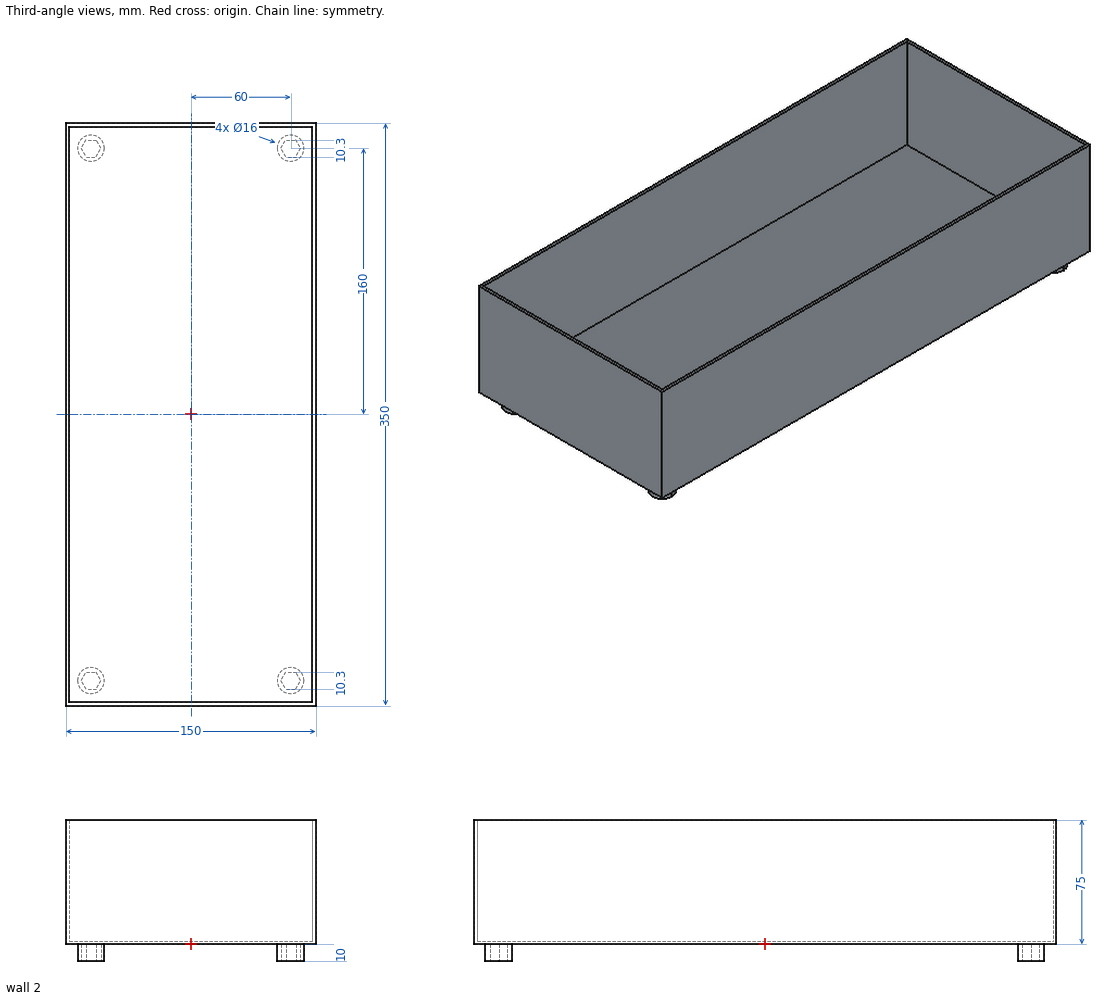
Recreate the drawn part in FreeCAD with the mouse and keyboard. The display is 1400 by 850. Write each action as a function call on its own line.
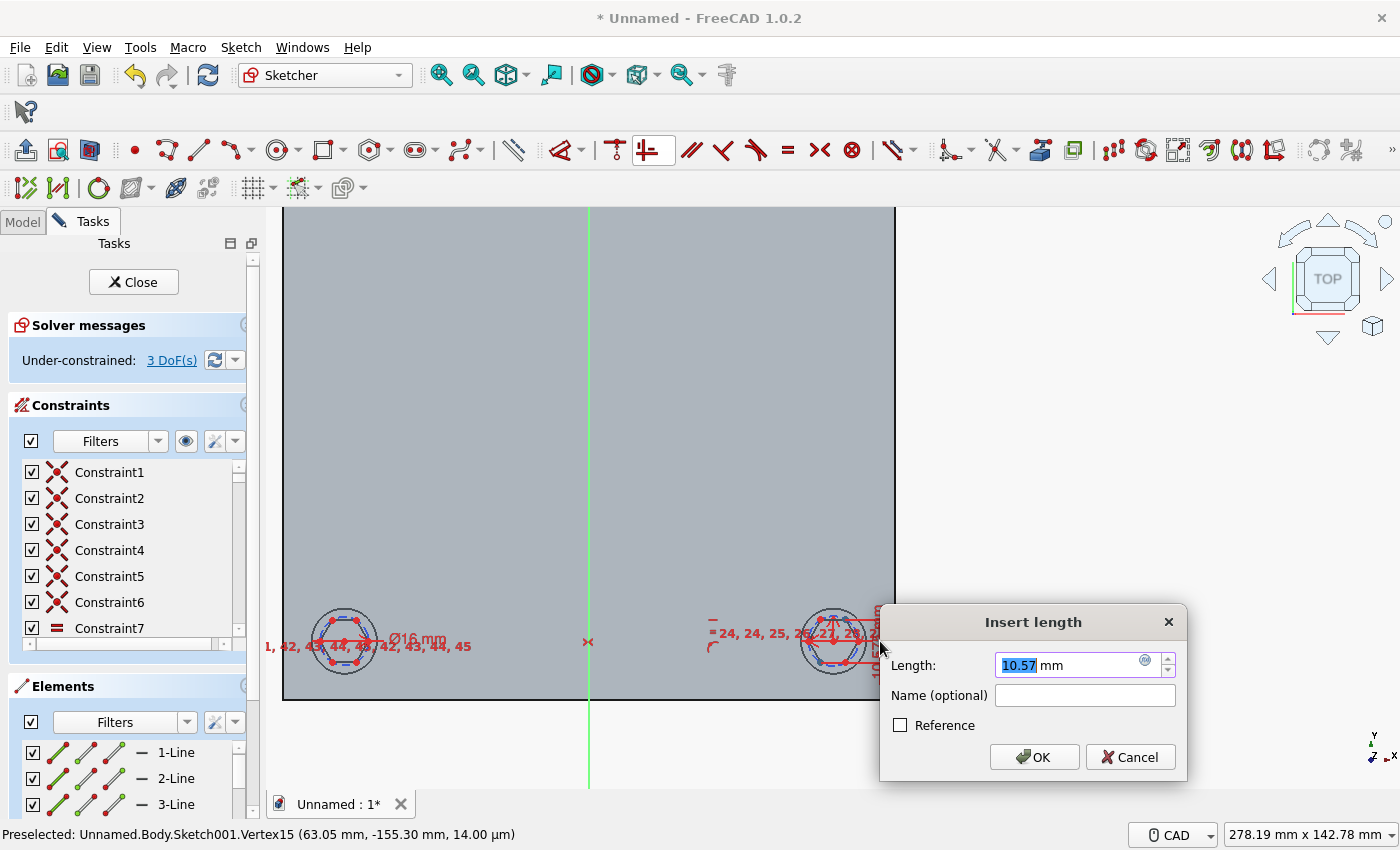
text(10.3)
key(Return)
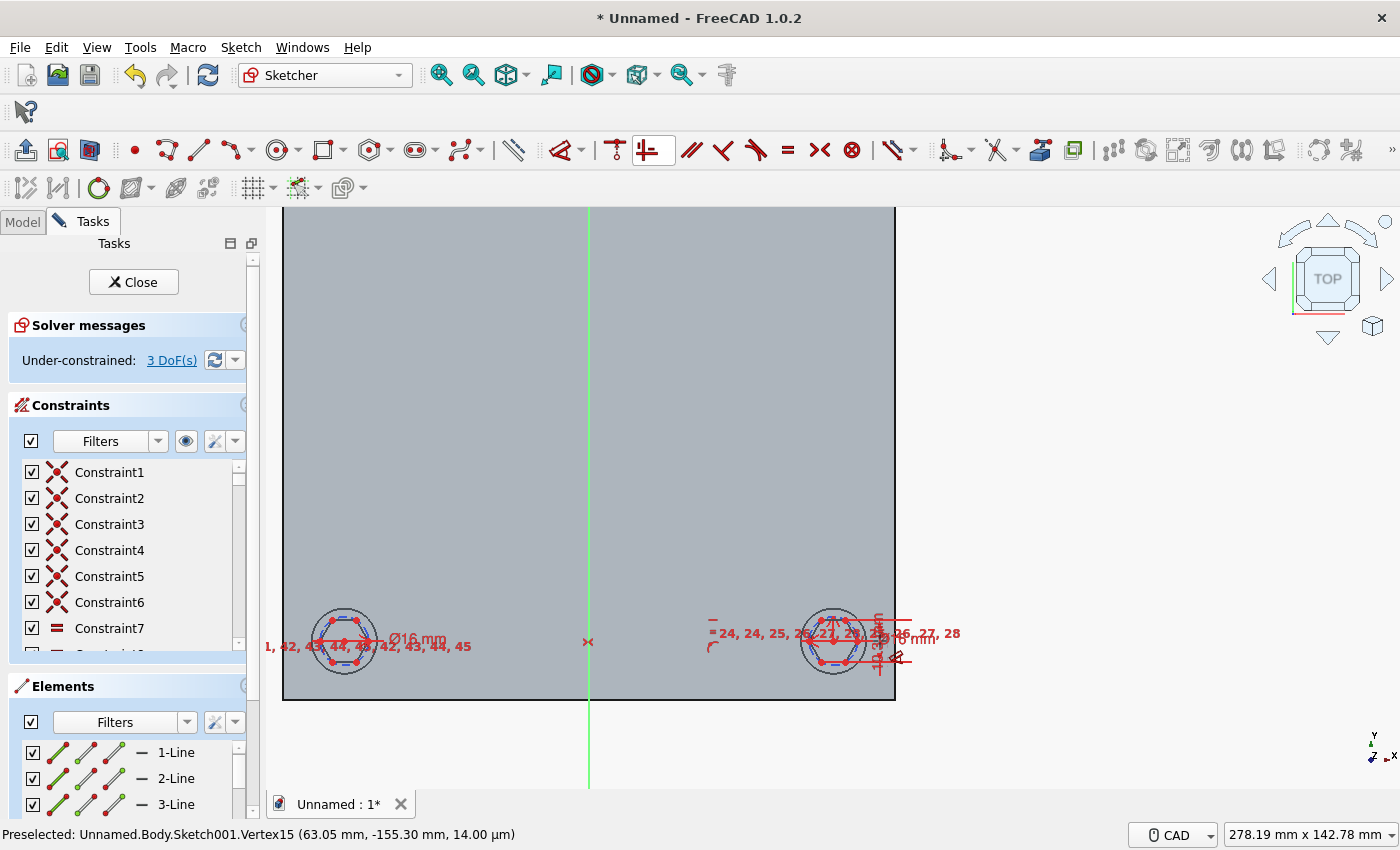
click(332, 662)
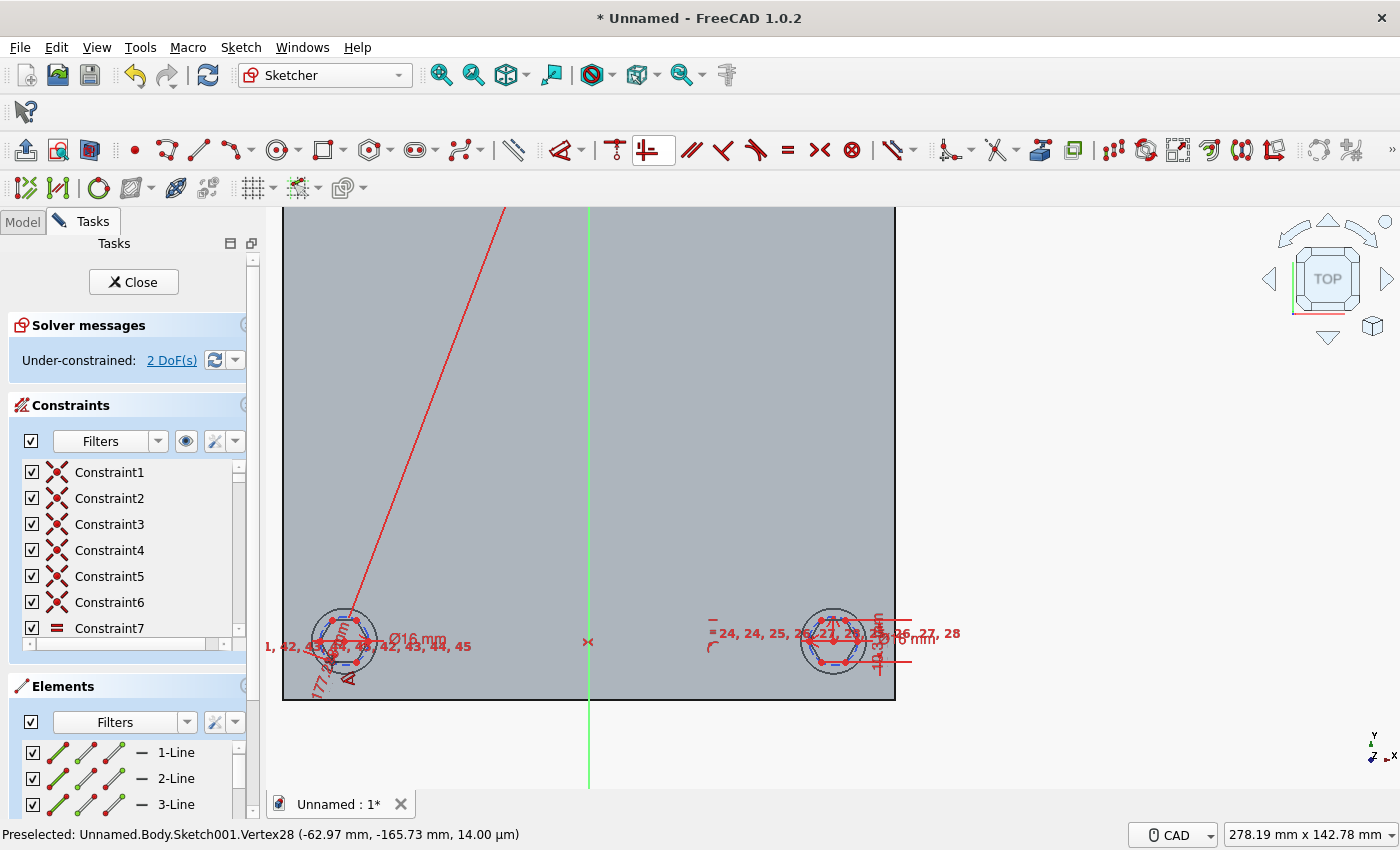
click(356, 620)
click(298, 641)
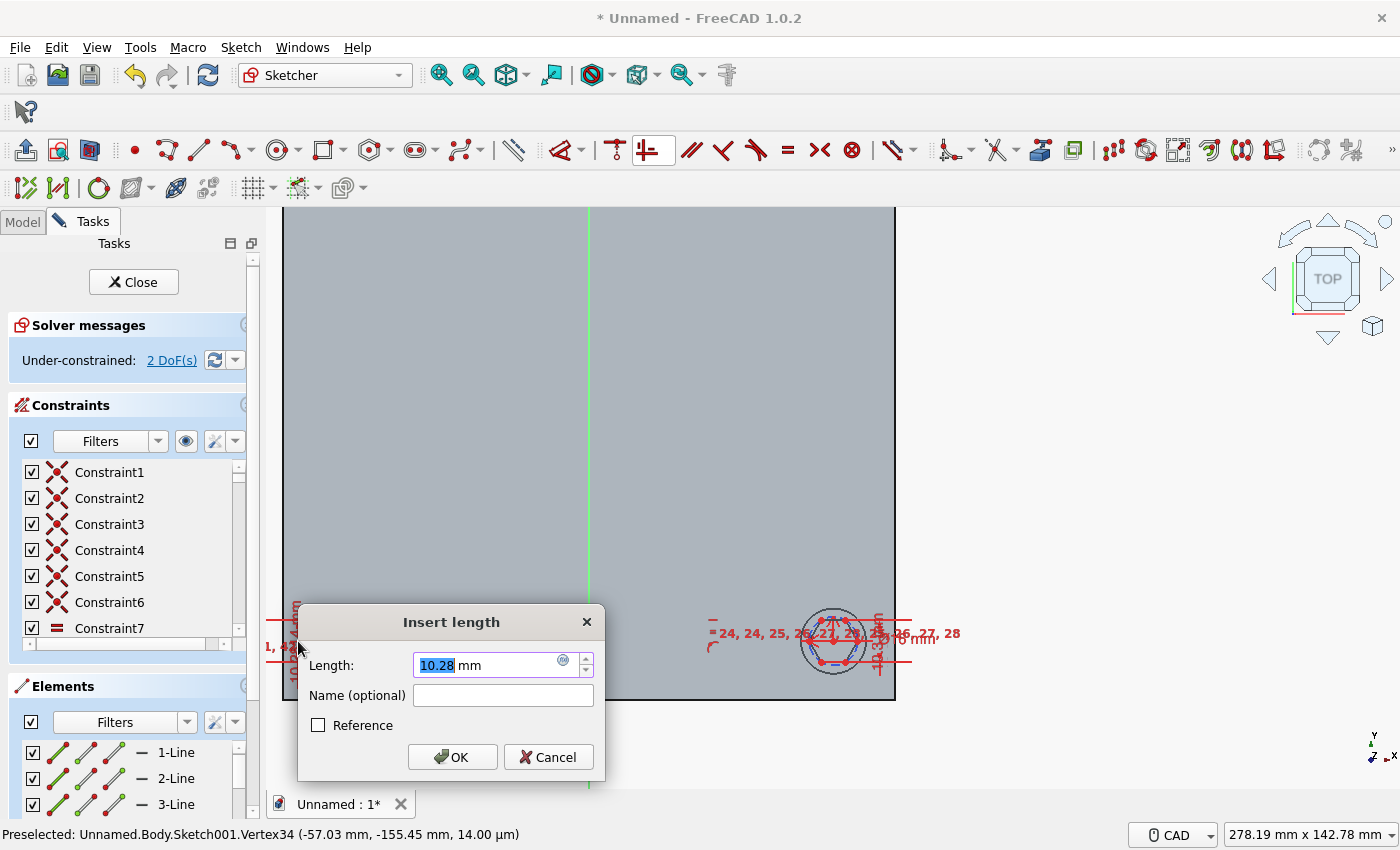
text(10.3)
key(Return)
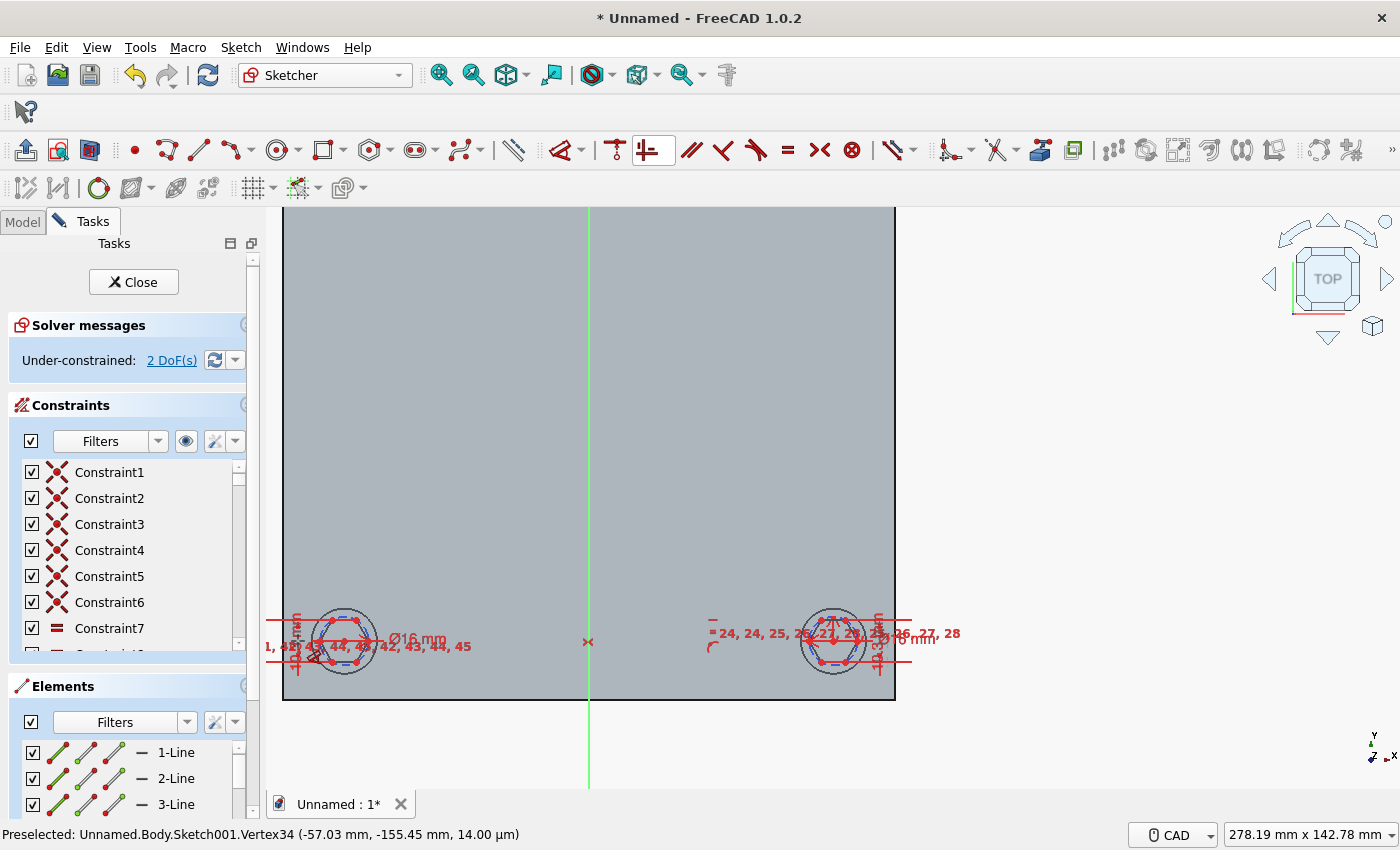
scroll(822, 665, down, 7)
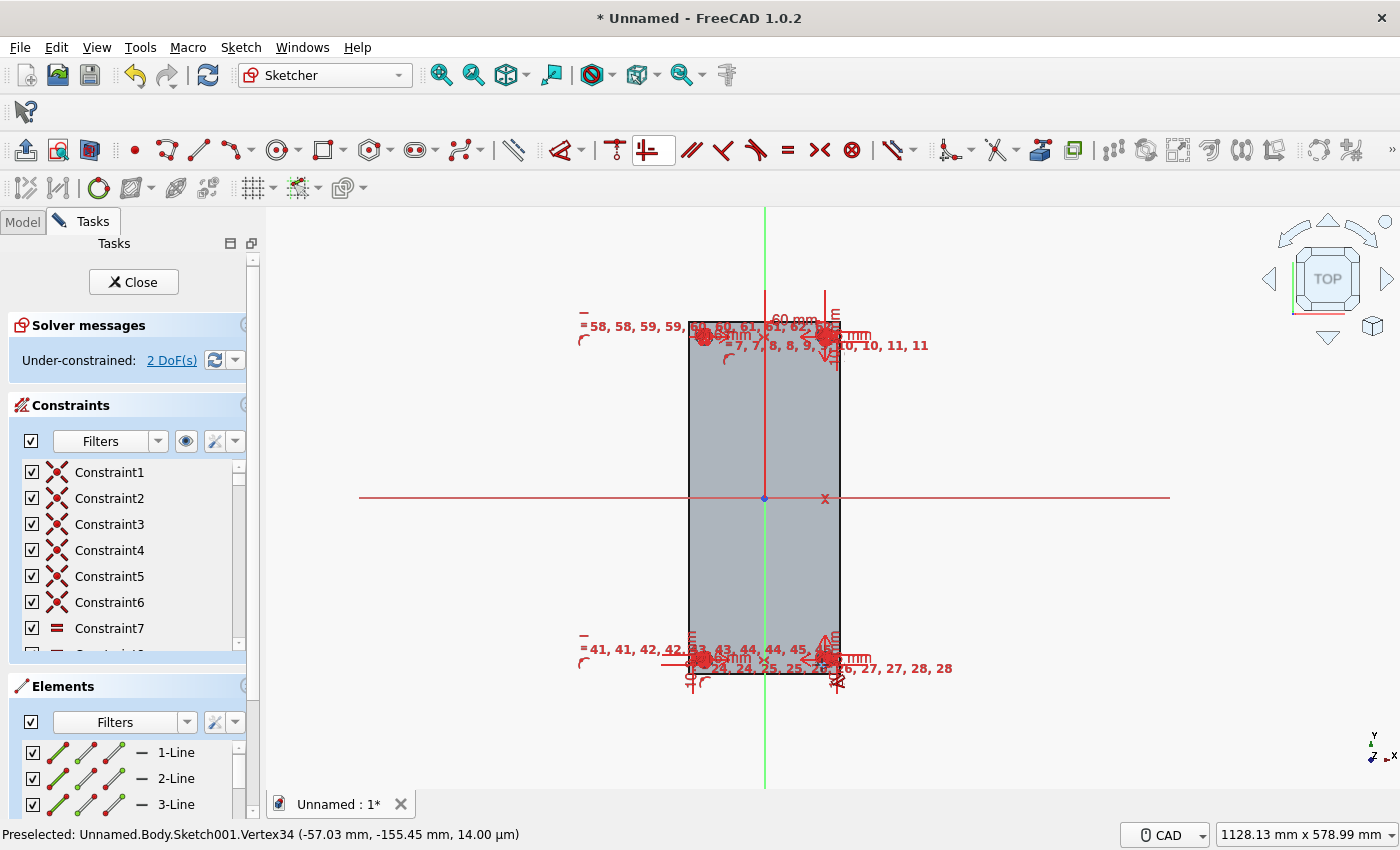
scroll(702, 342, up, 7)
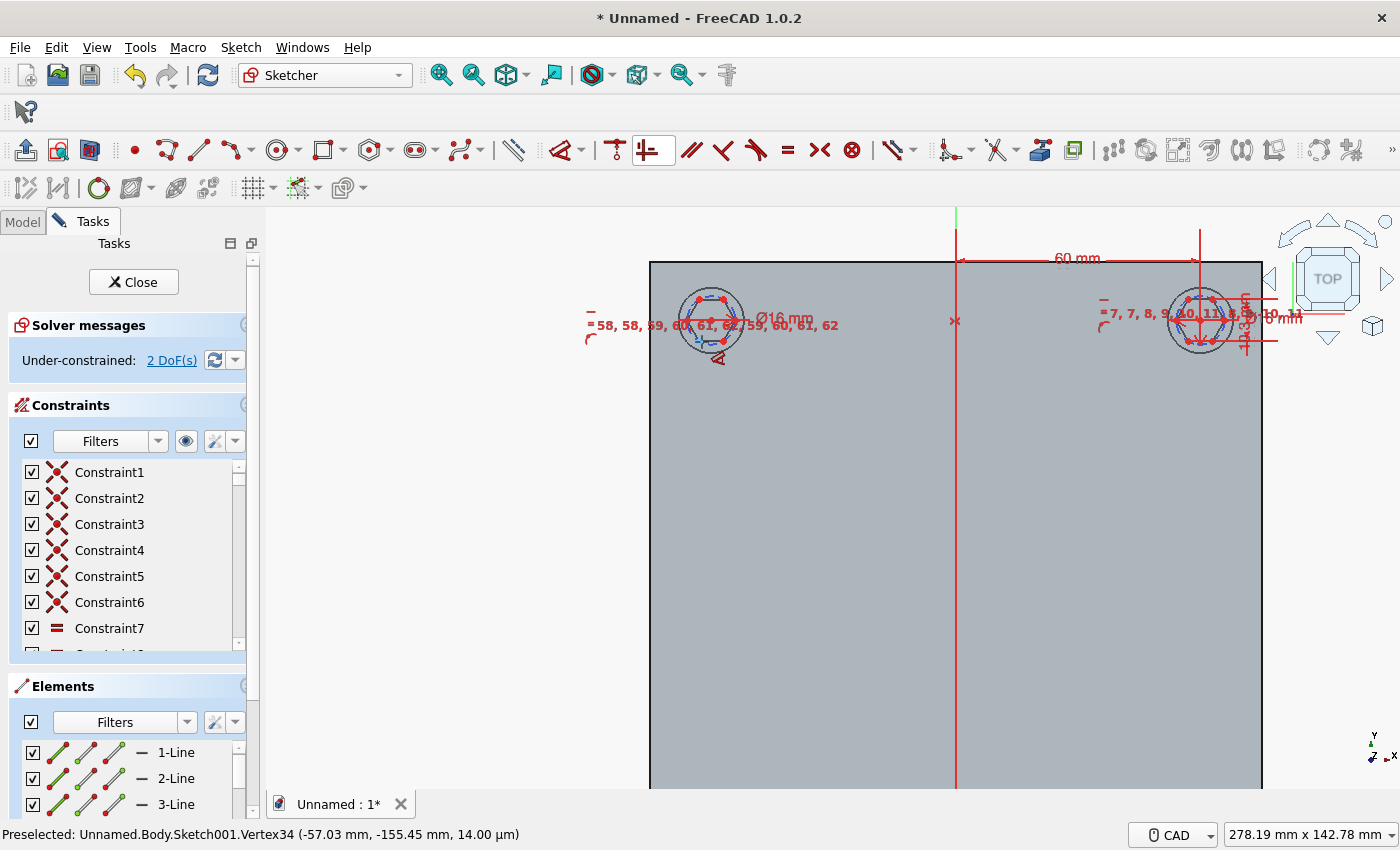
click(699, 341)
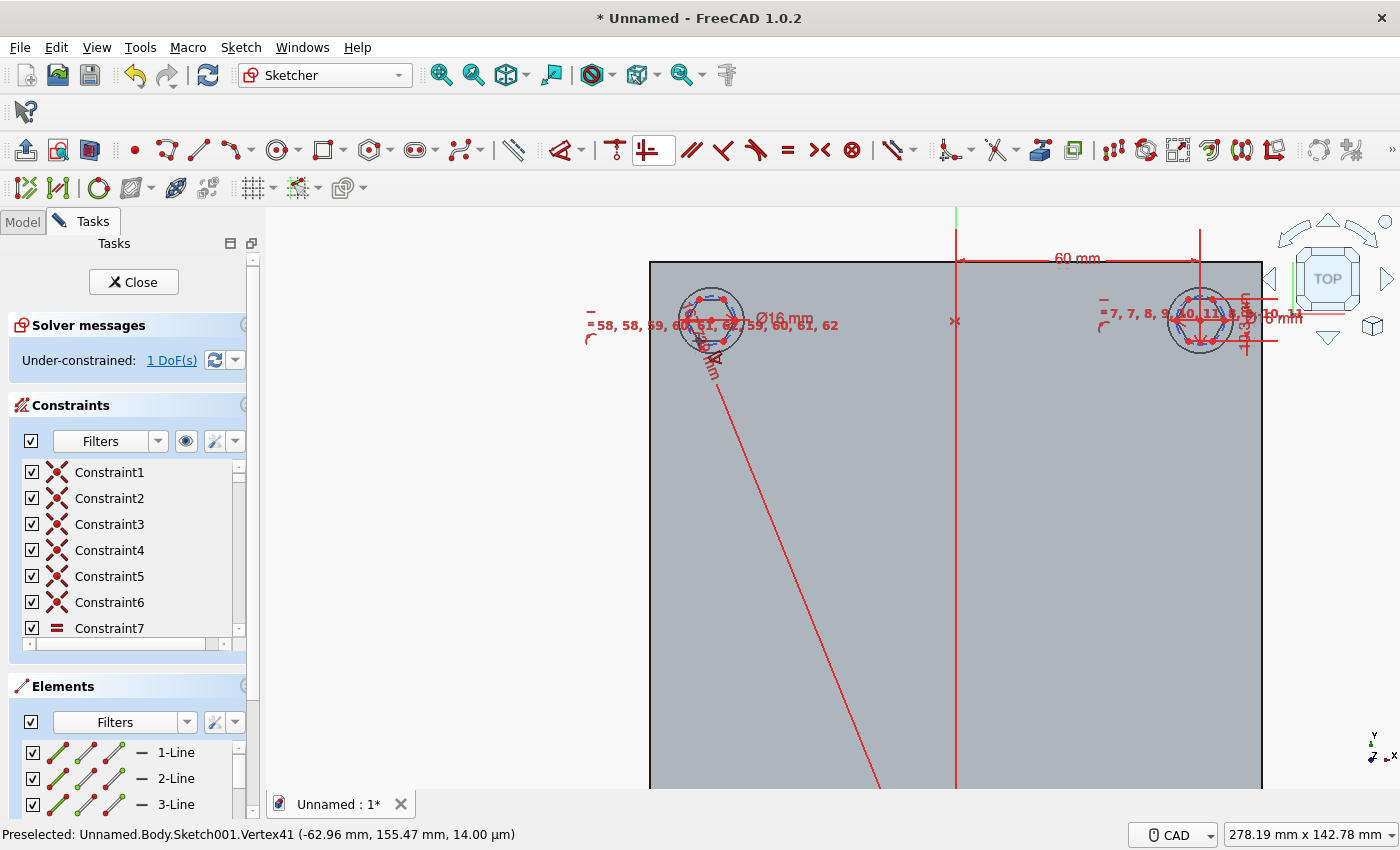
click(723, 300)
click(665, 320)